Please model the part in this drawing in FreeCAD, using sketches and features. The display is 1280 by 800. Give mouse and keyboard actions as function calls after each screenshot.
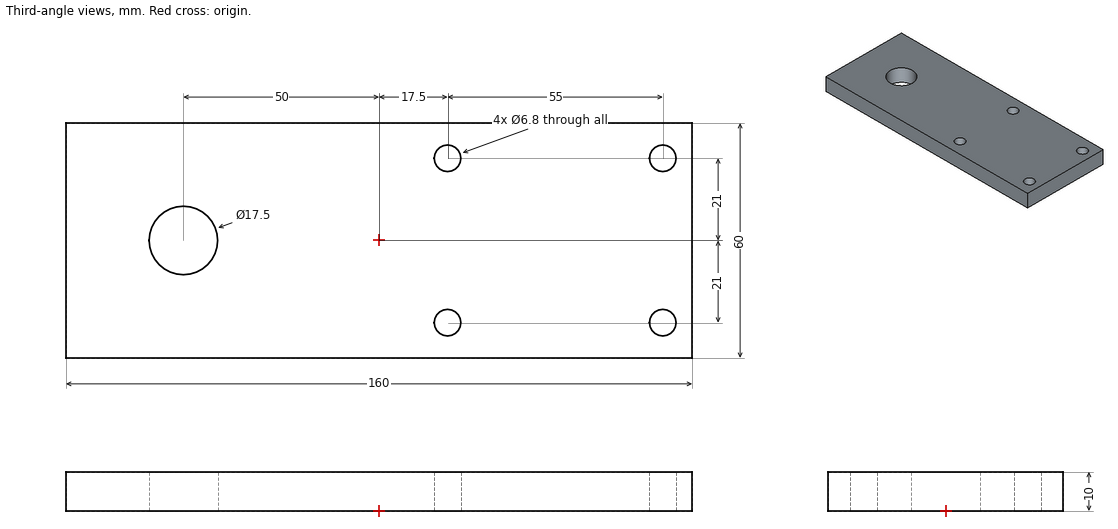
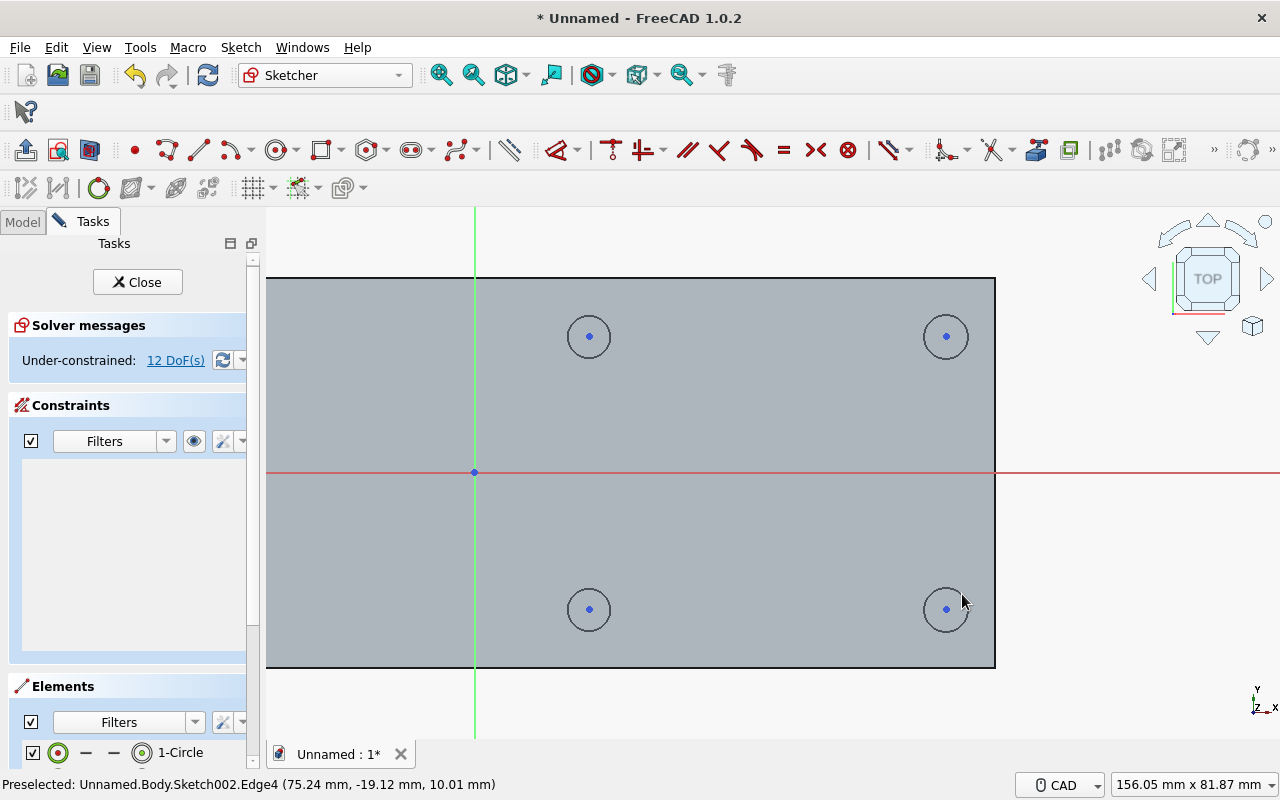
click(604, 322)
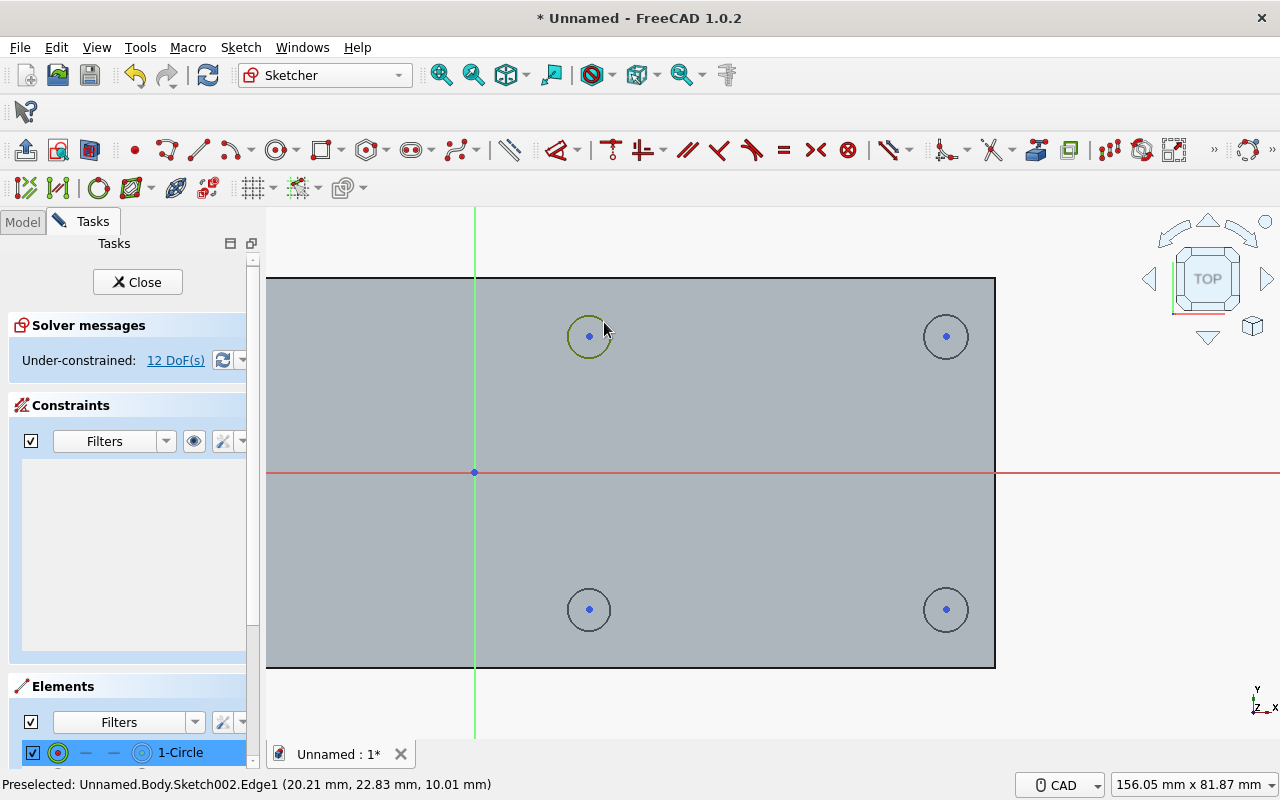
click(961, 321)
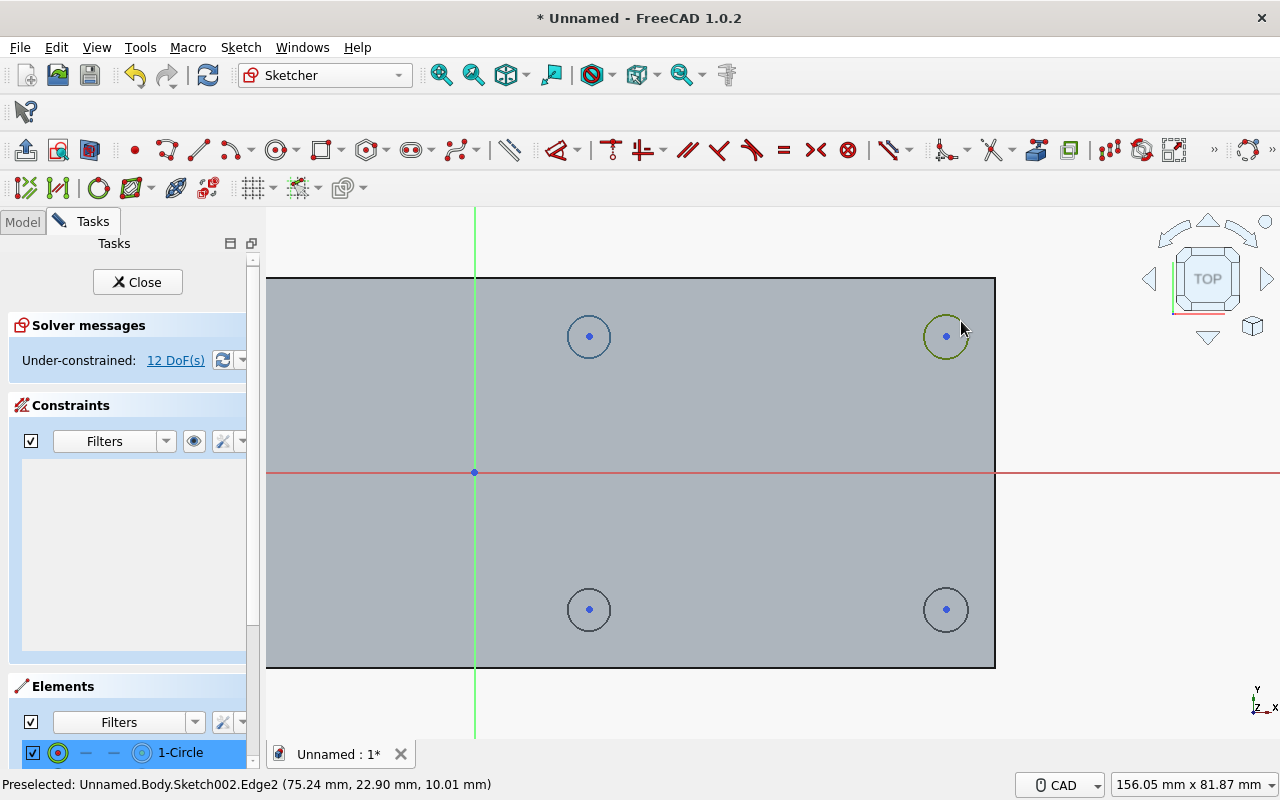
click(604, 595)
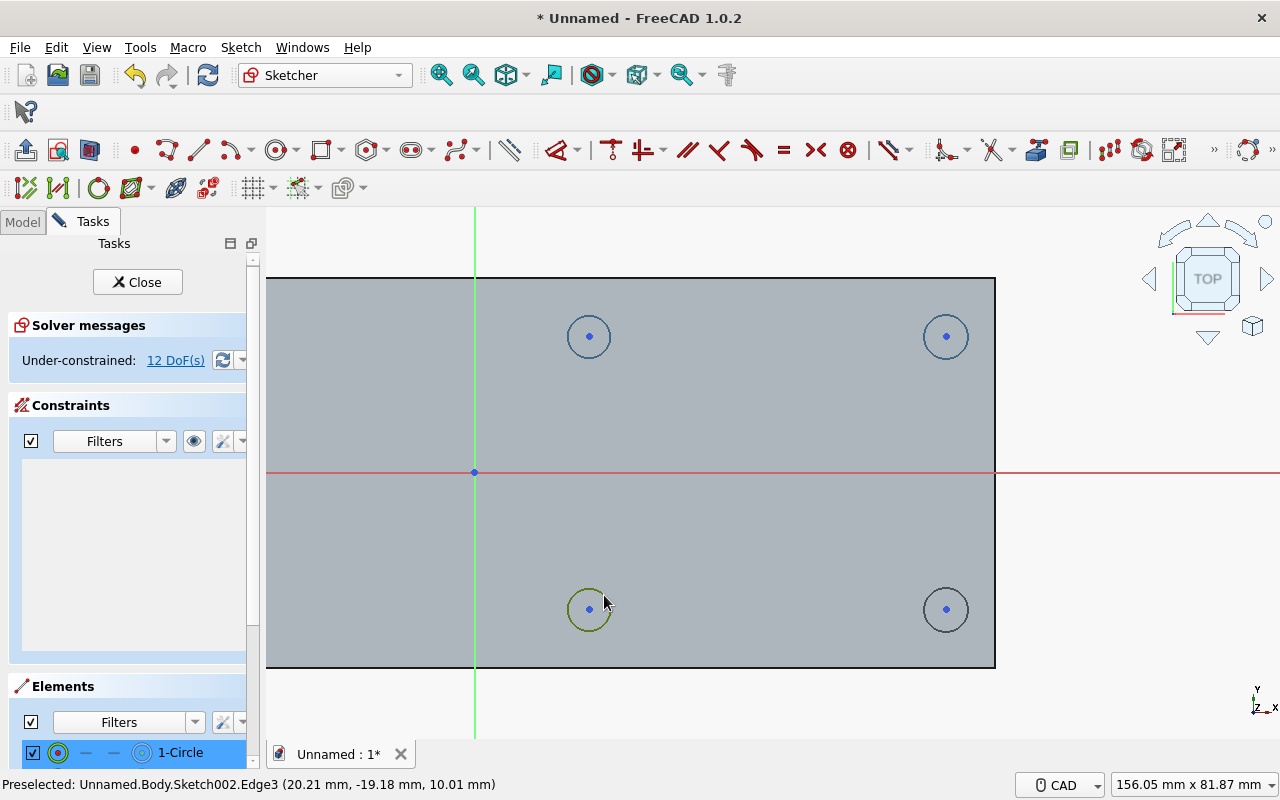
click(961, 594)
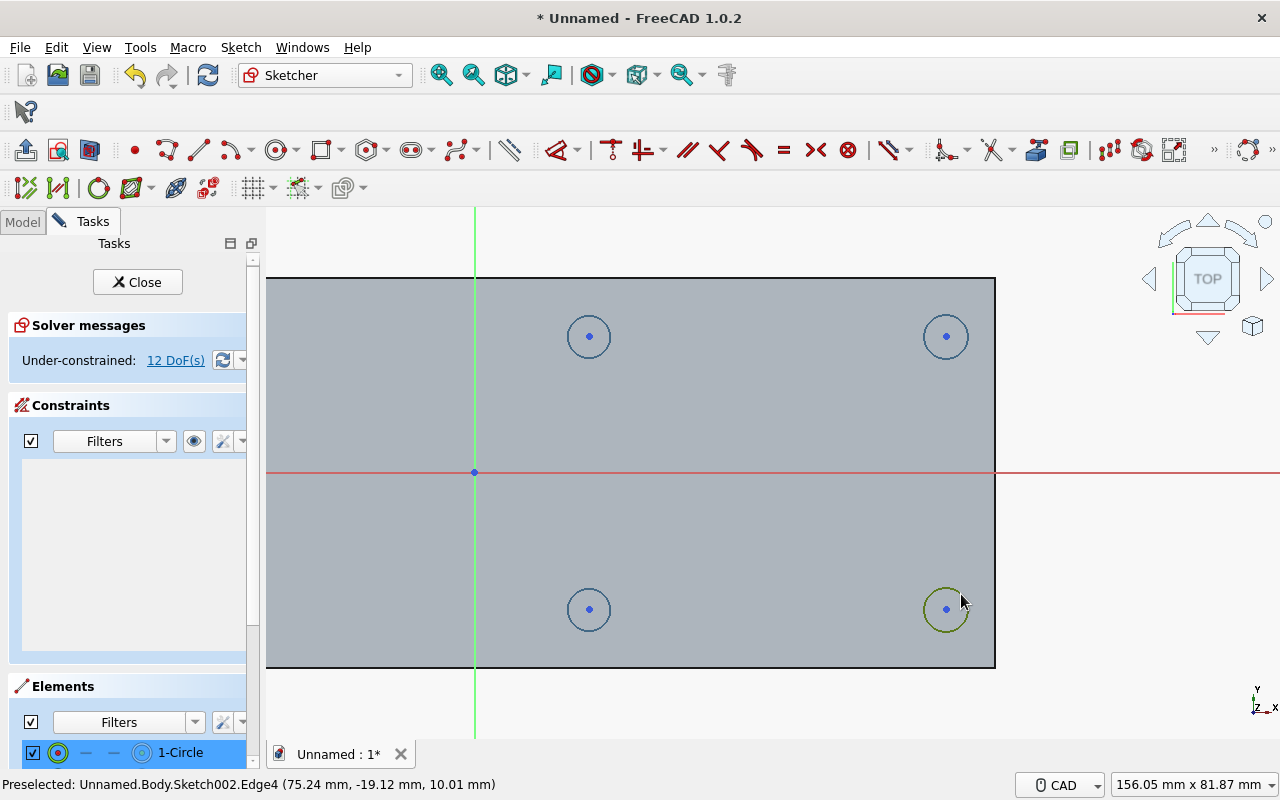
key(e)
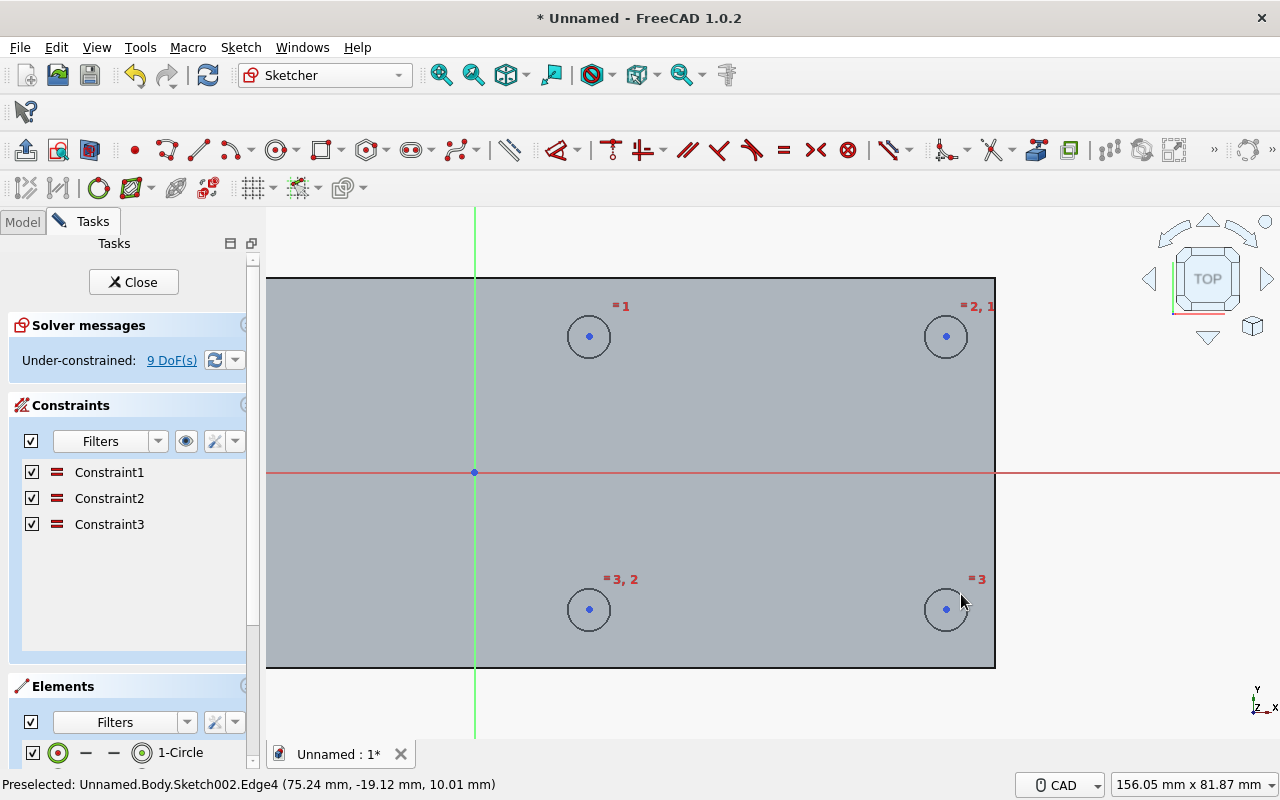
click(589, 337)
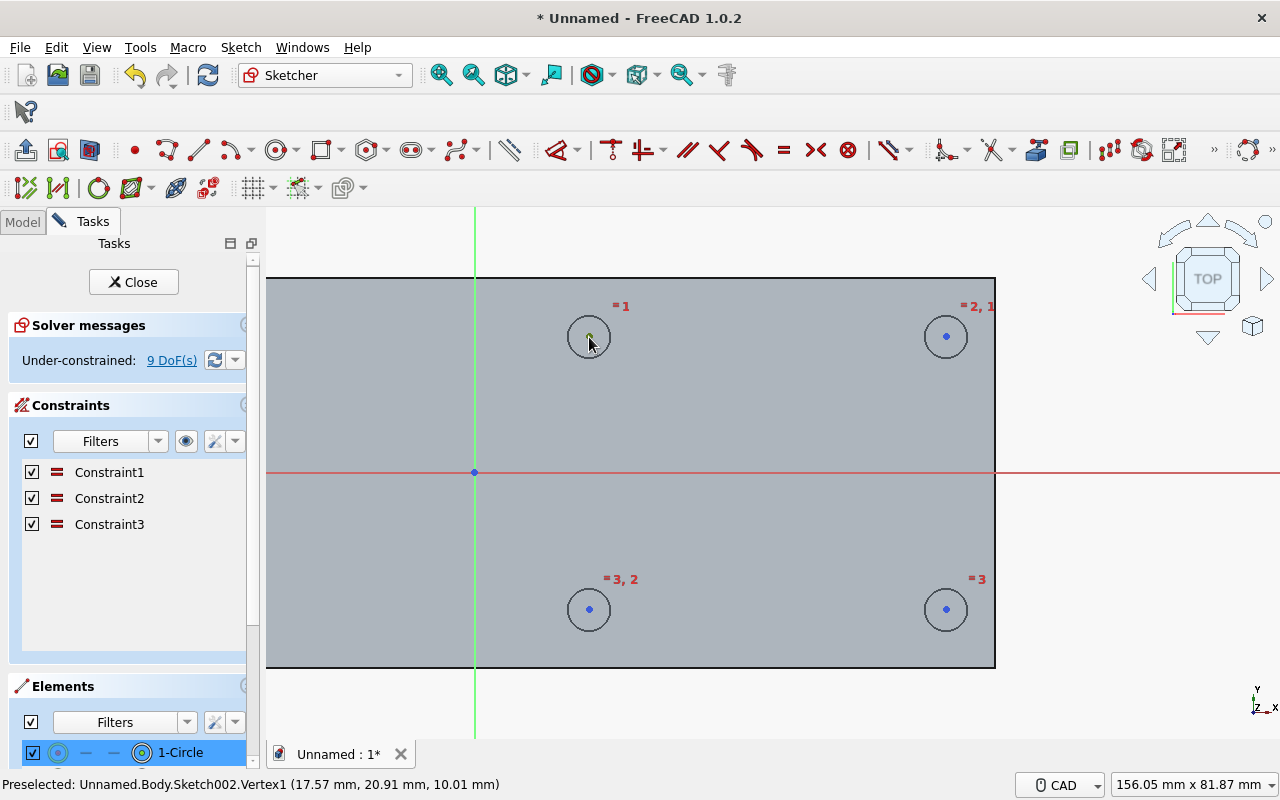
click(946, 337)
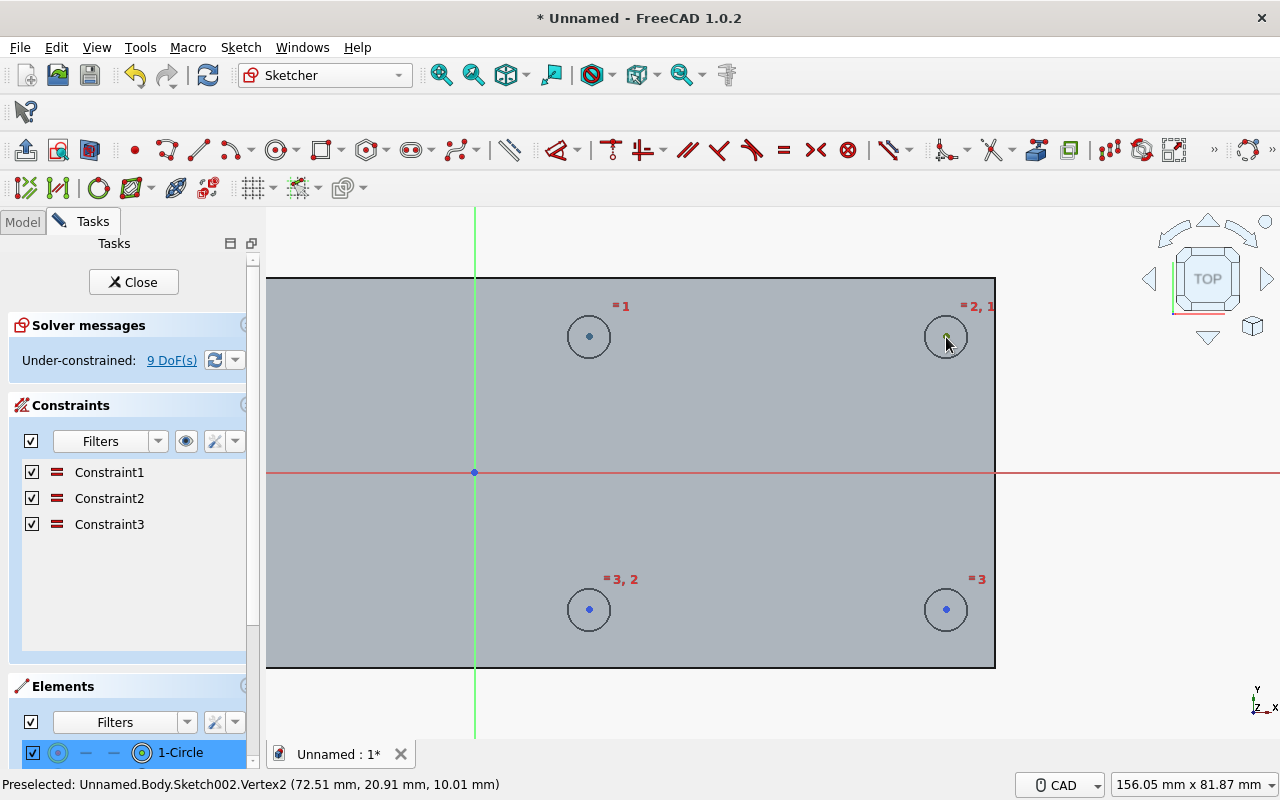
key(h)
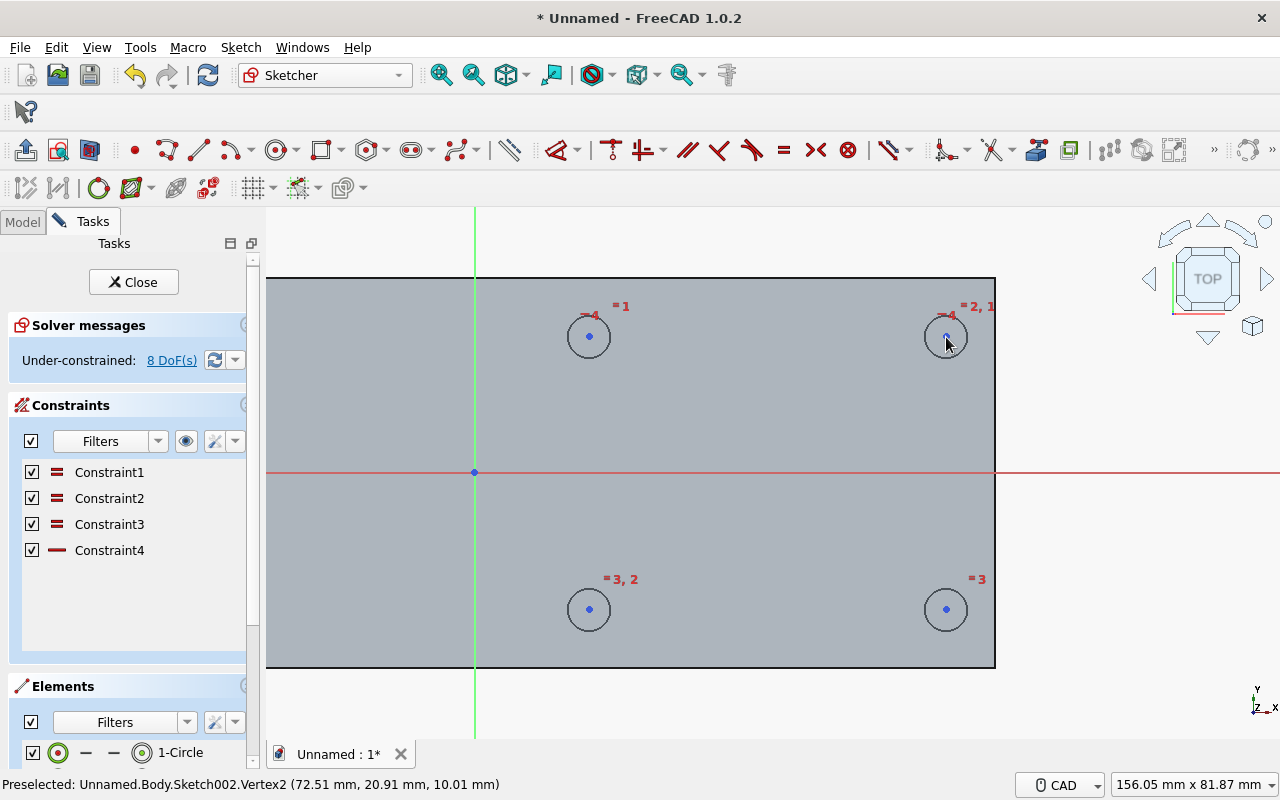
click(589, 337)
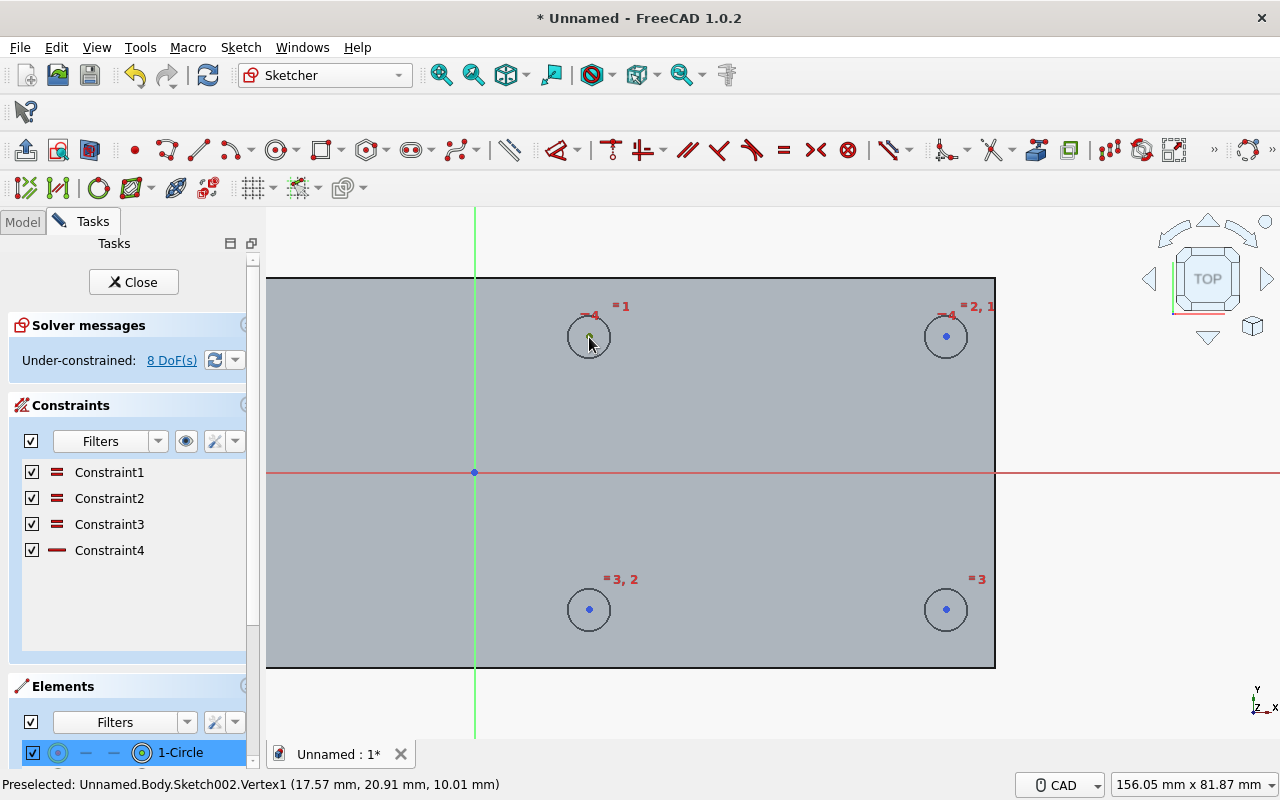
click(589, 610)